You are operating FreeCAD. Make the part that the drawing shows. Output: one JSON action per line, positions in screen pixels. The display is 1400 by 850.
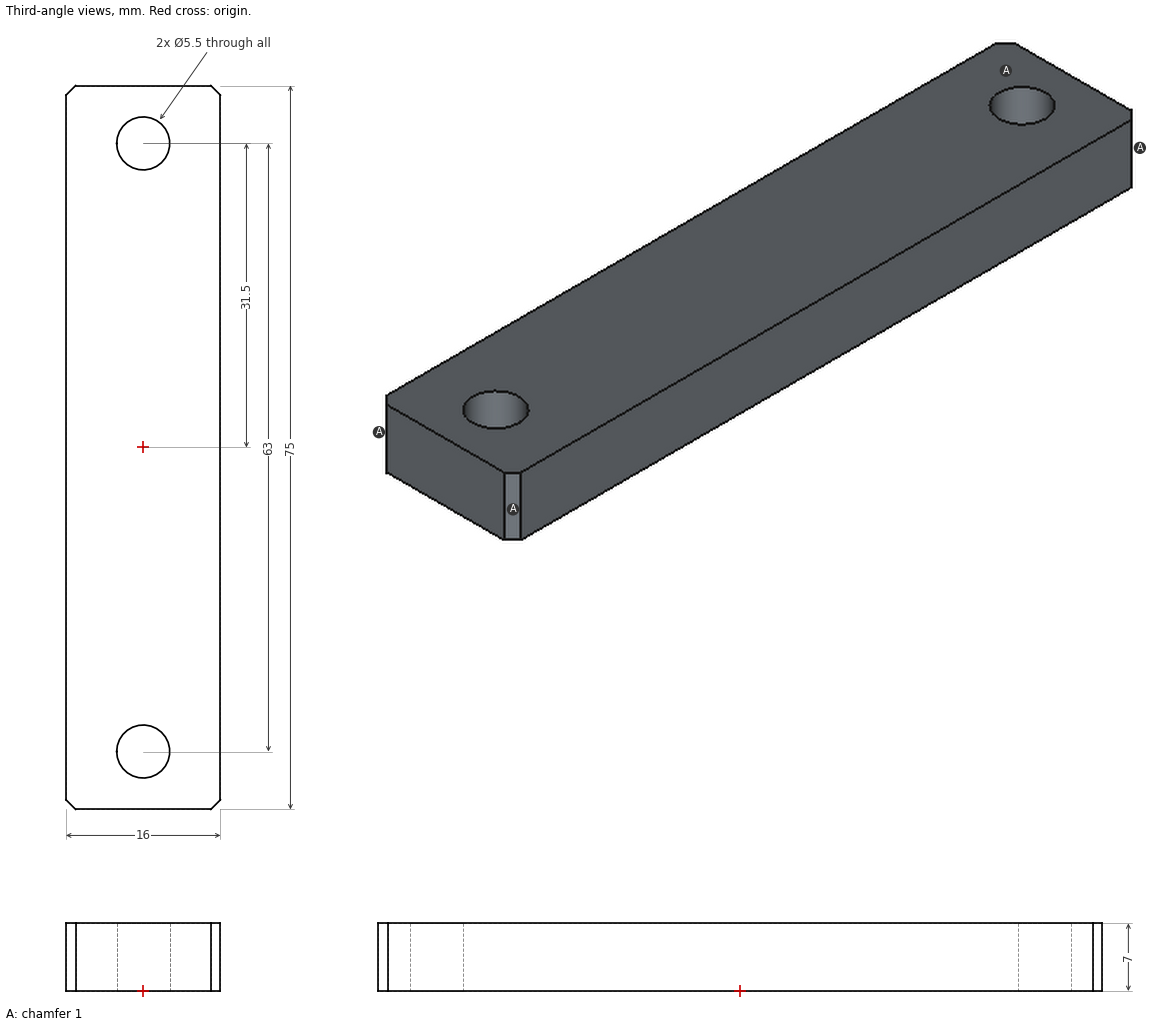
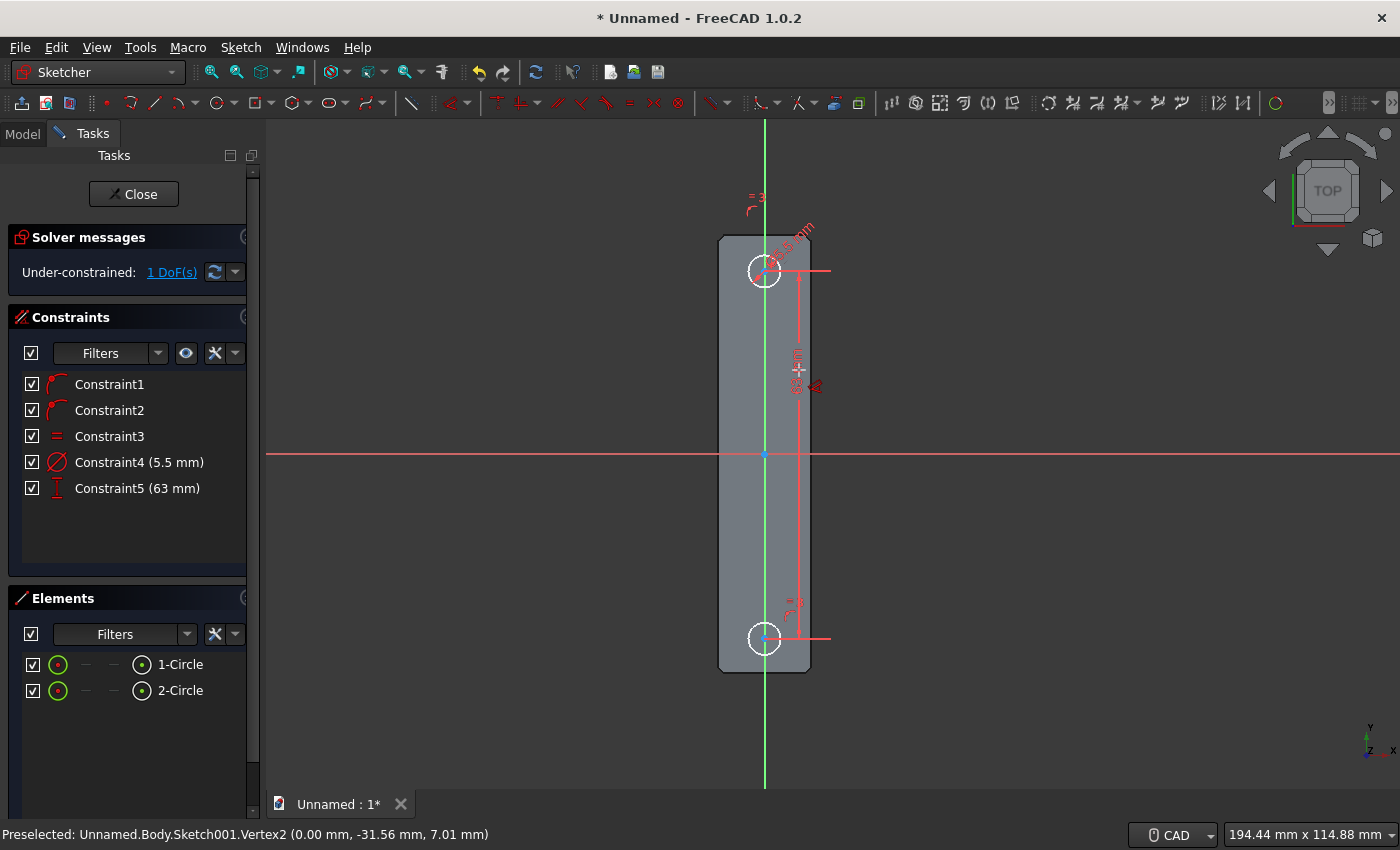
{"action": "left_click", "coordinate": [765, 271]}
{"action": "left_click", "coordinate": [799, 321]}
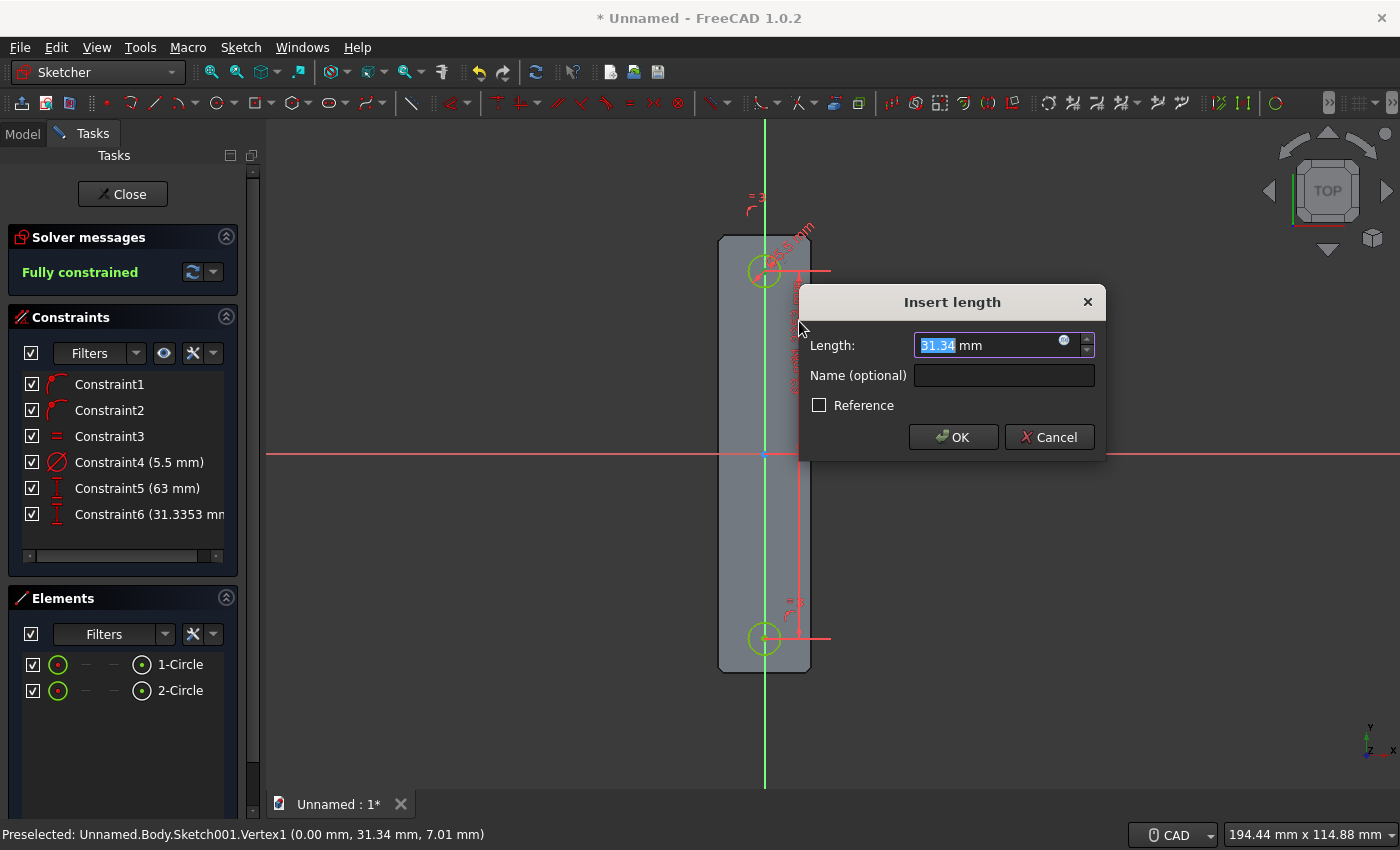
{"action": "type", "text": "31.5"}
{"action": "key", "text": "Return"}
{"action": "key", "text": "Escape"}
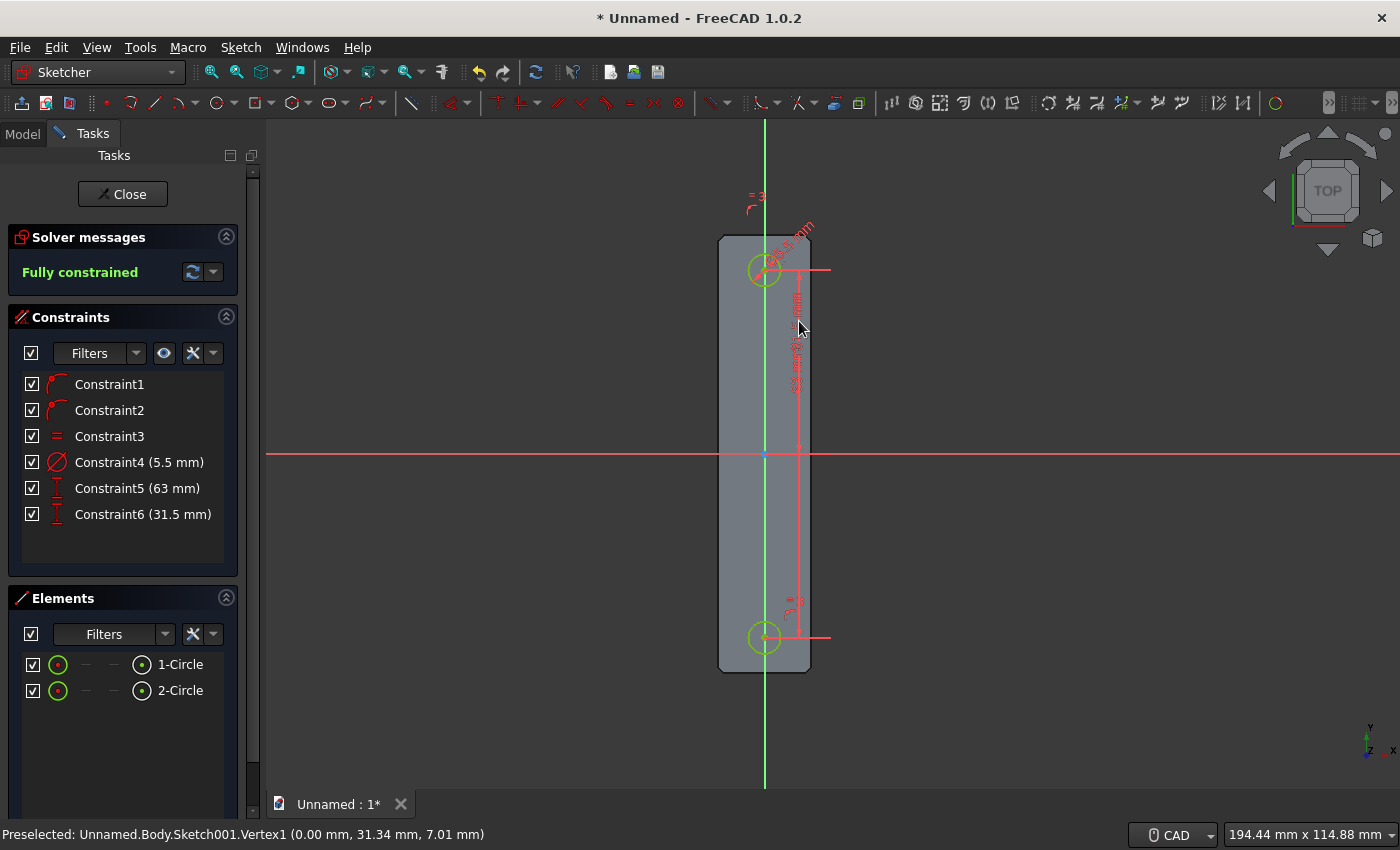
{"action": "left_click", "coordinate": [123, 194]}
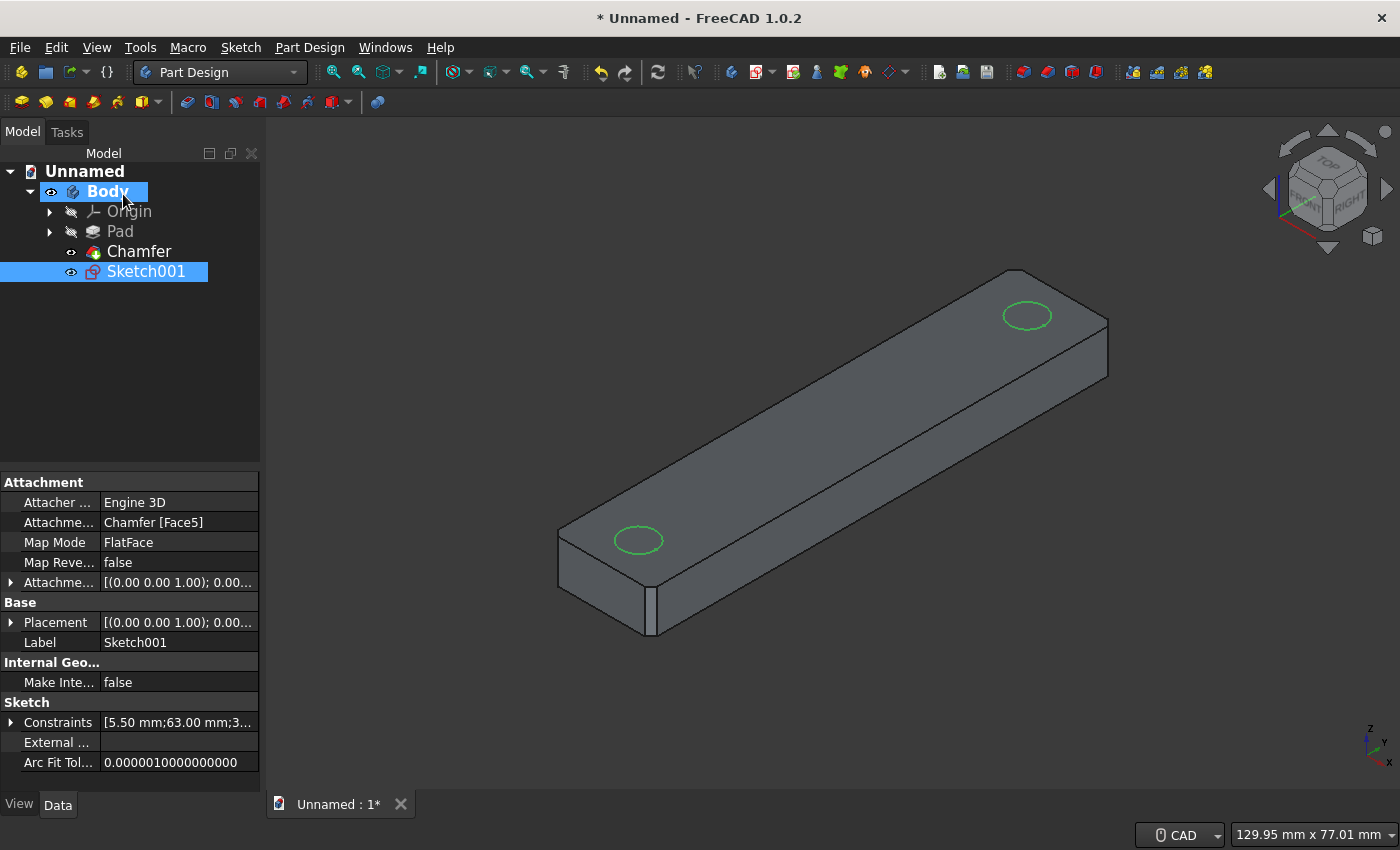
{"action": "left_click", "coordinate": [212, 102]}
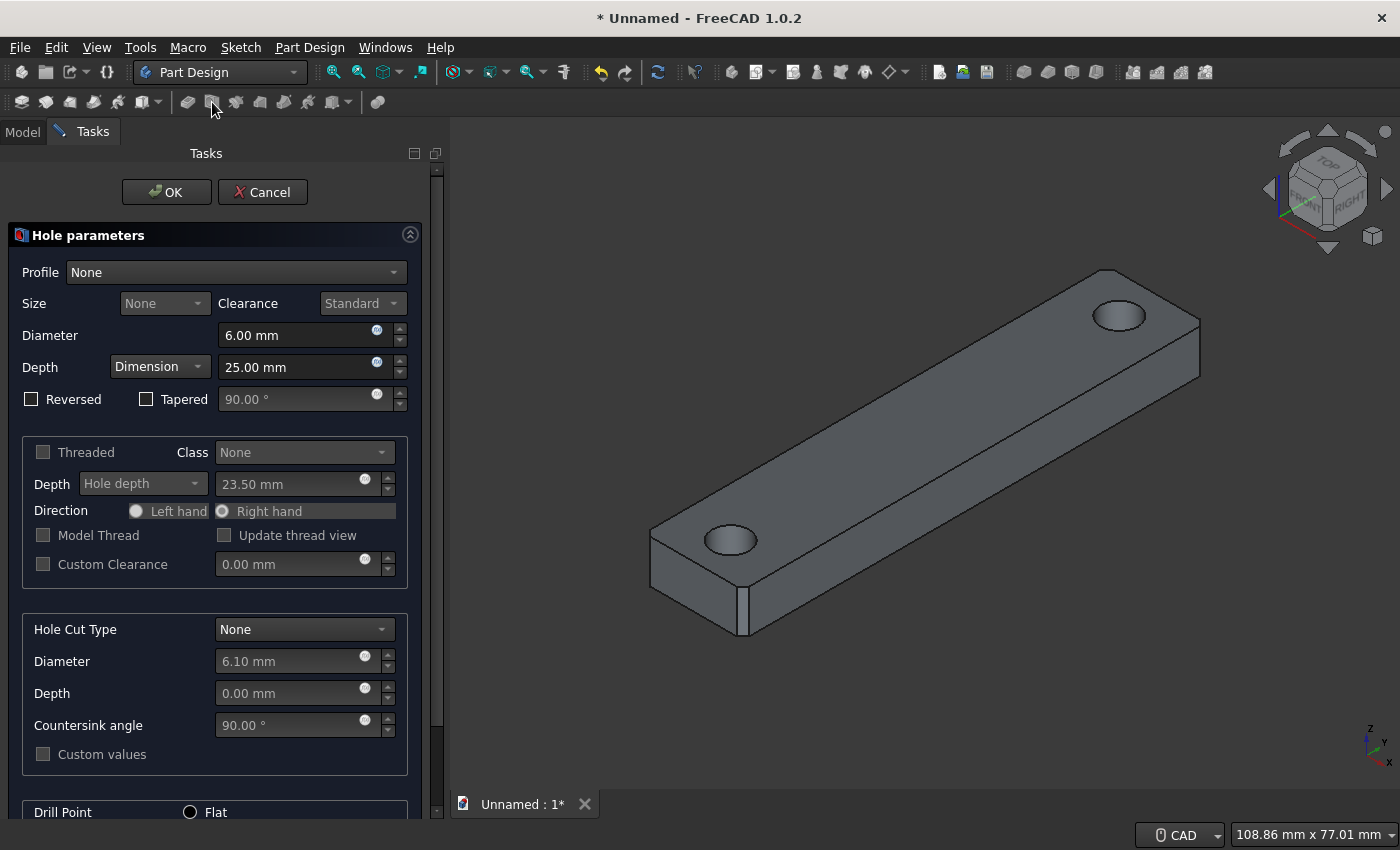
{"action": "triple_click", "coordinate": [305, 335]}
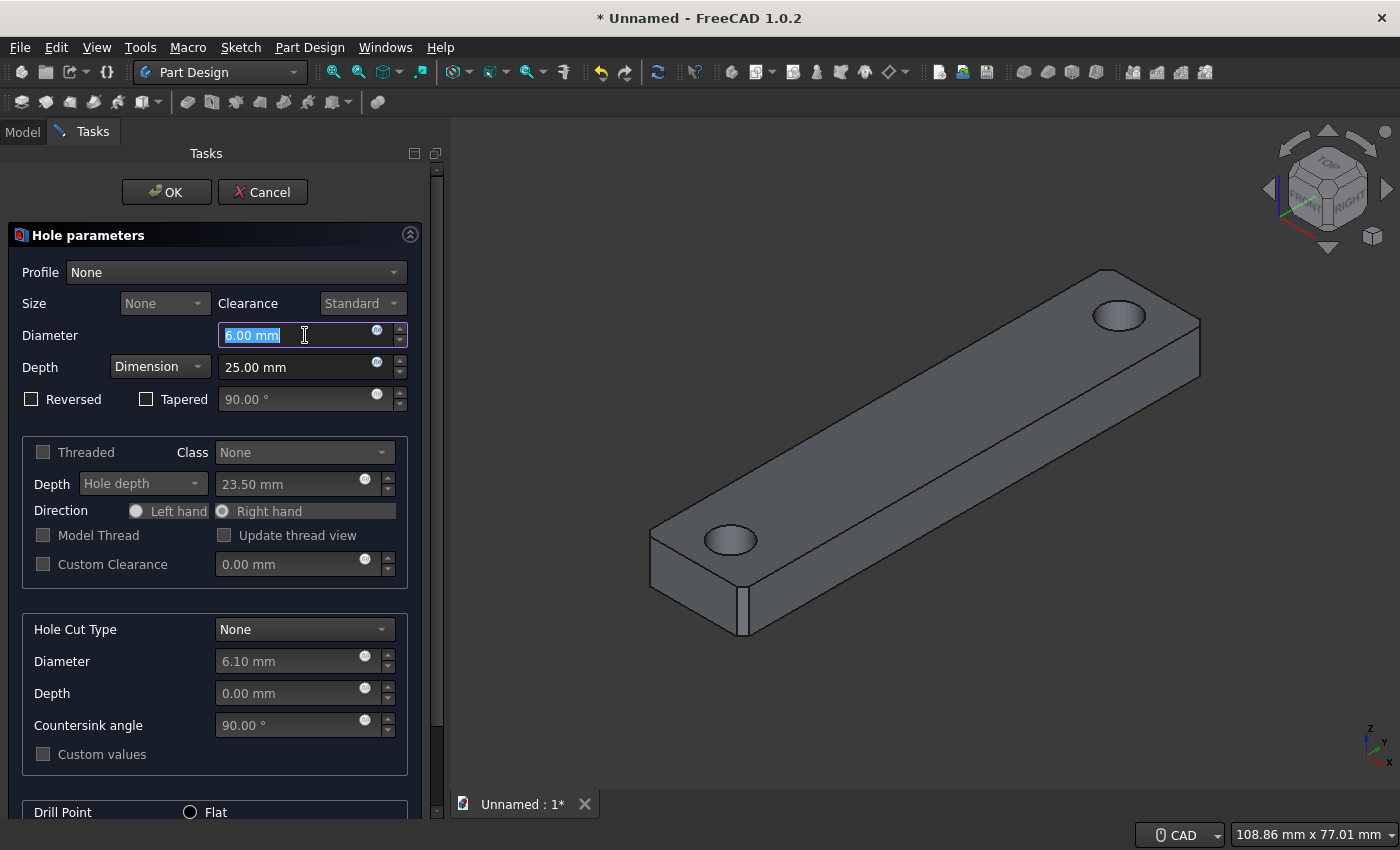
{"action": "type", "text": "5.5"}
{"action": "key", "text": "Tab"}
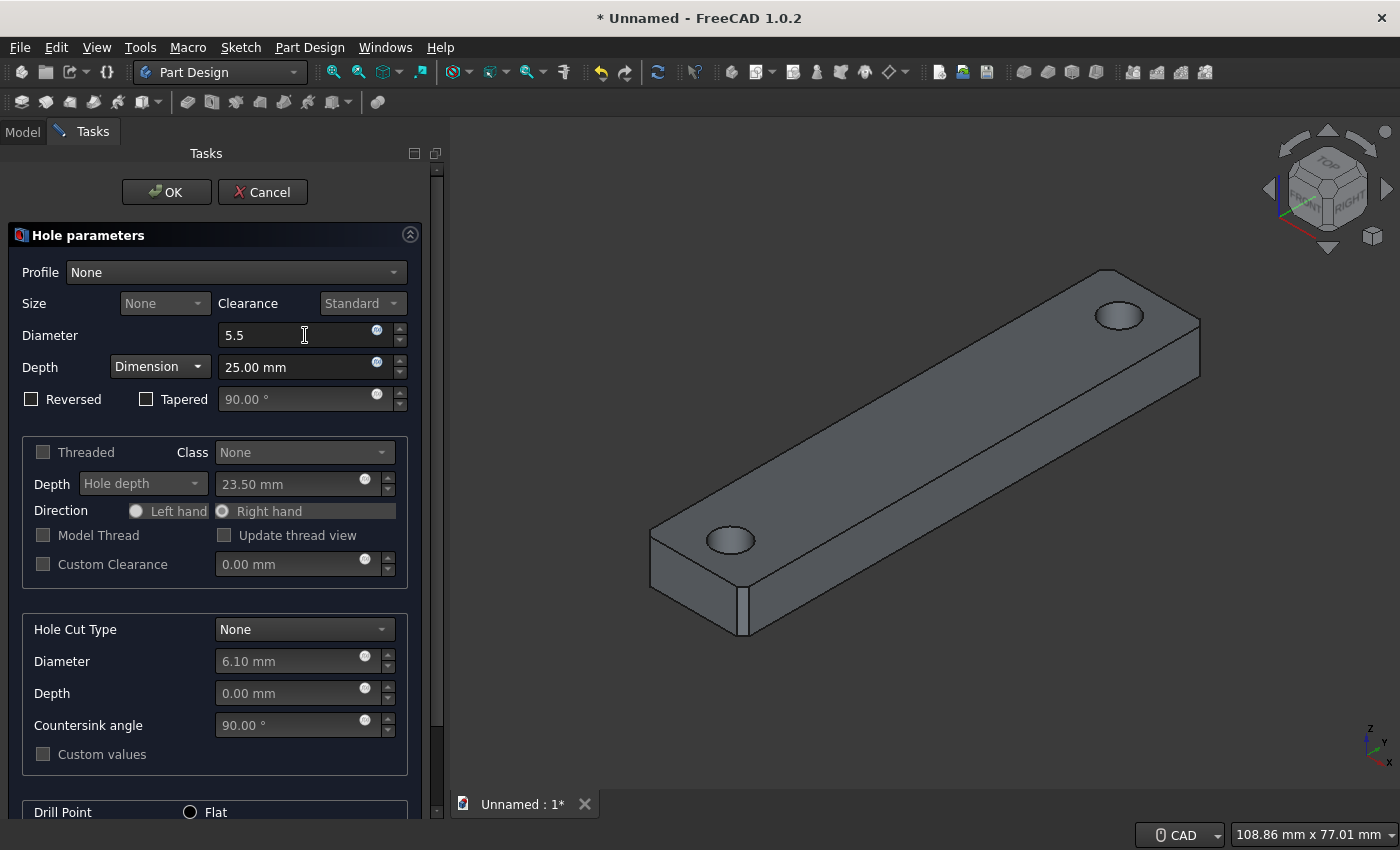
{"action": "left_click", "coordinate": [161, 366]}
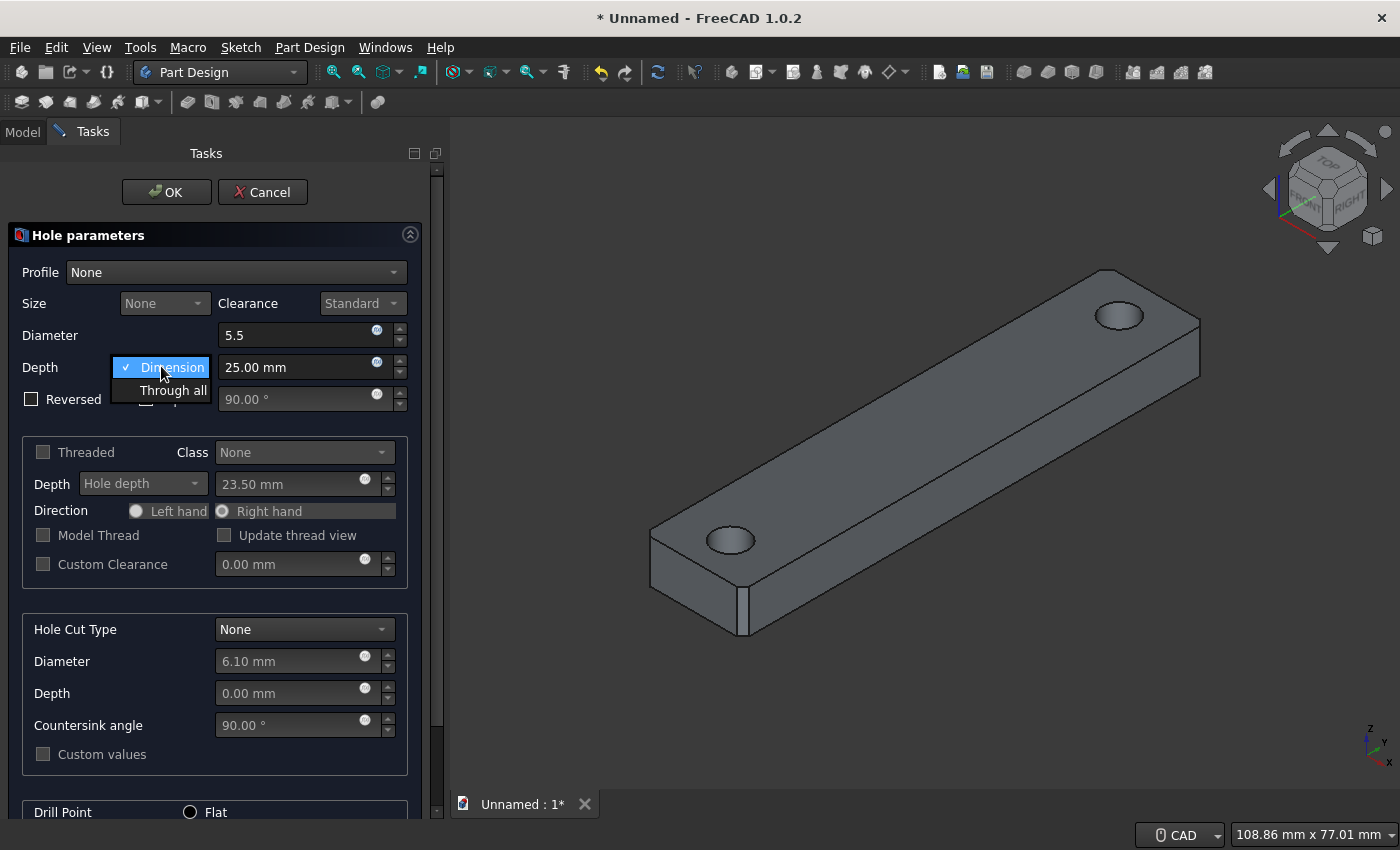
{"action": "left_click", "coordinate": [160, 390]}